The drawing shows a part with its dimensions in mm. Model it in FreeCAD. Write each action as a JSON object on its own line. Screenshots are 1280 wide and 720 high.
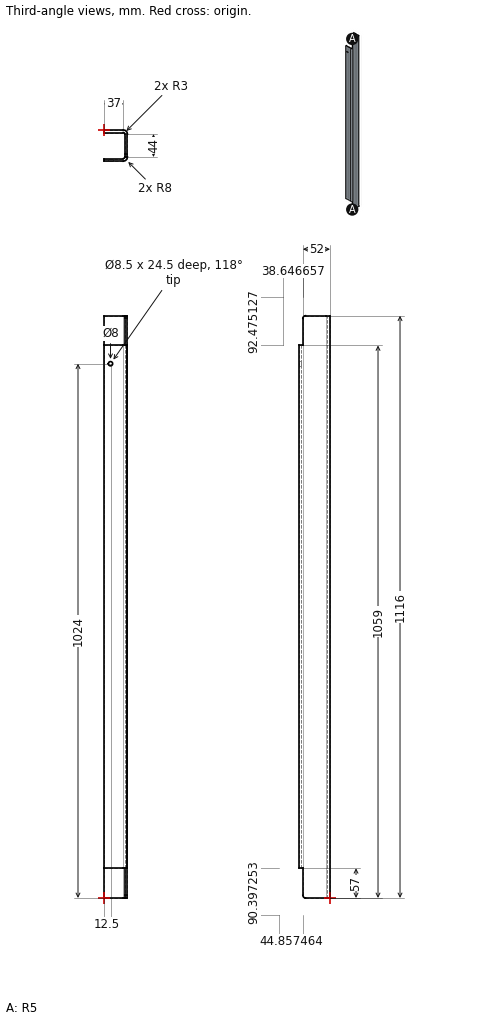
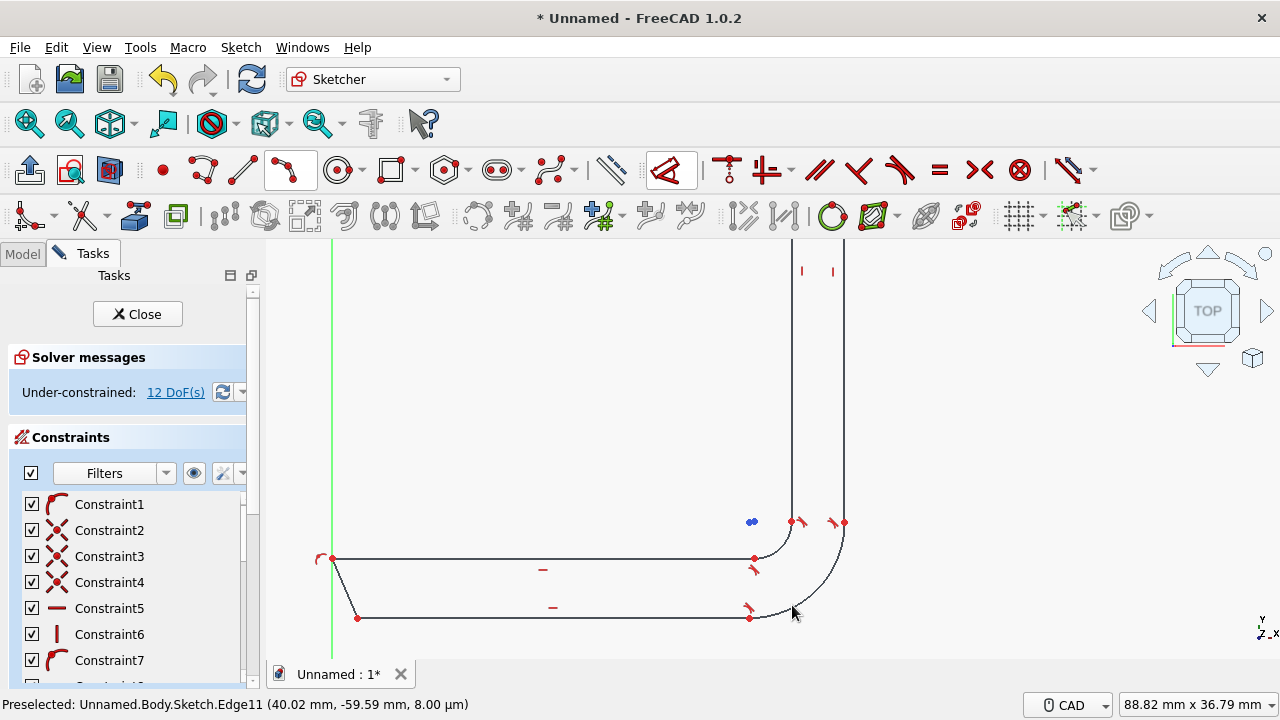
{"action": "left_click", "coordinate": [844, 372]}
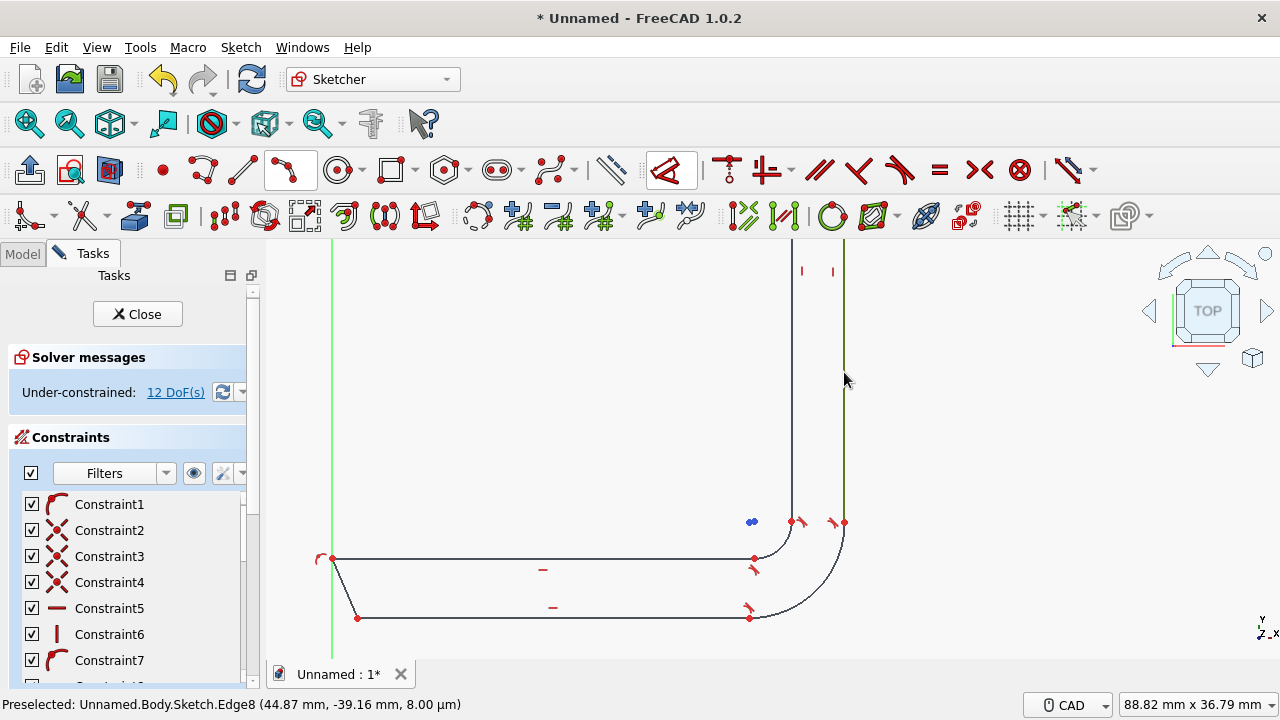
{"action": "scroll", "coordinate": [772, 554], "scroll_direction": "down", "scroll_amount": 5}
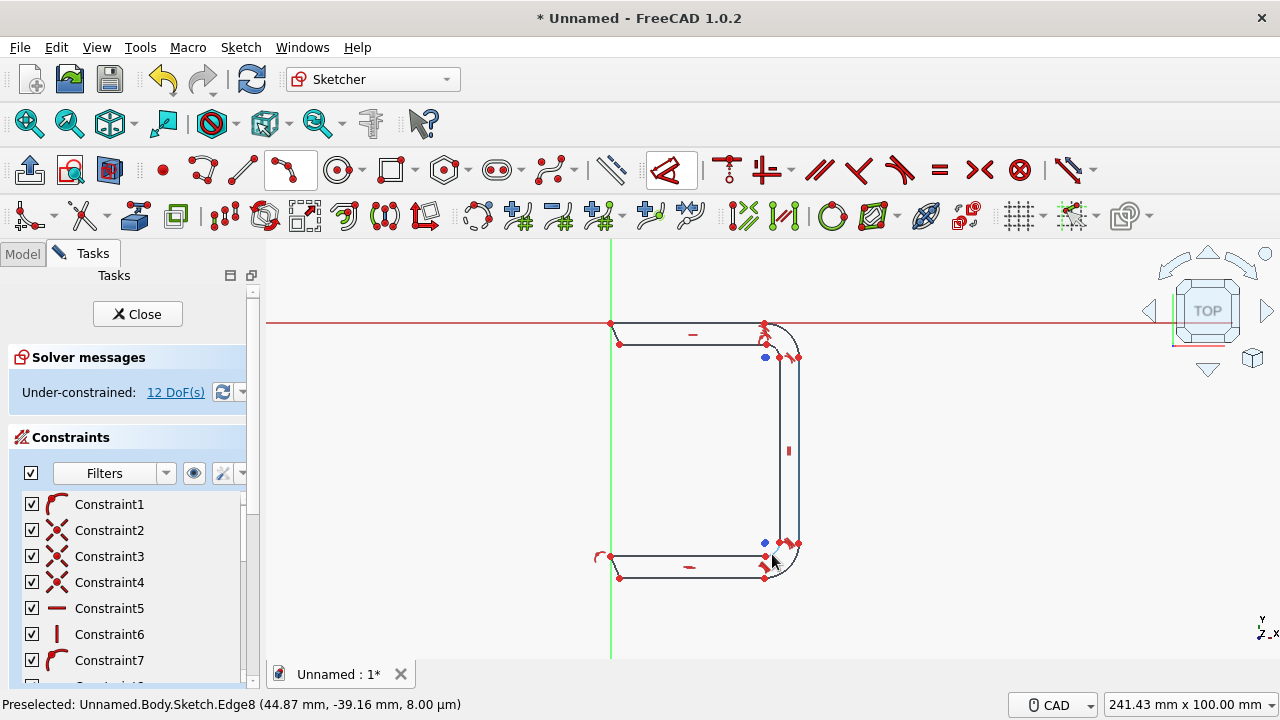
{"action": "left_click", "coordinate": [795, 342]}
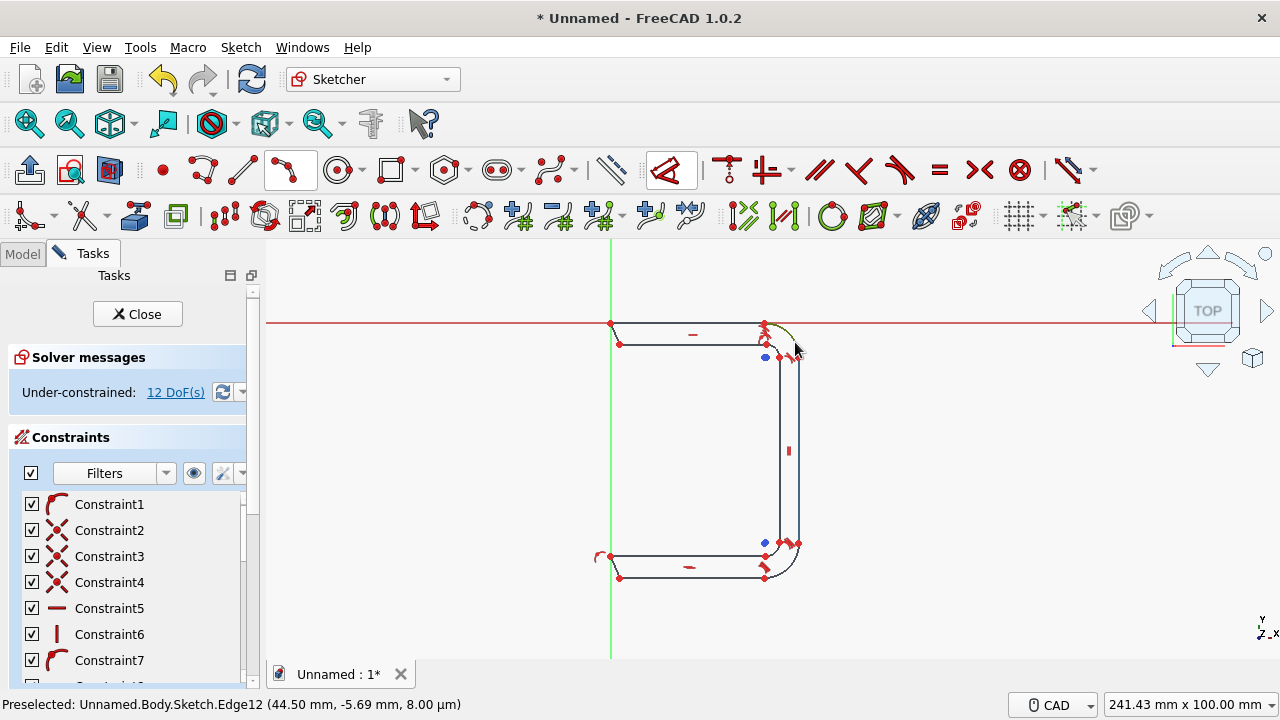
{"action": "key", "text": "t"}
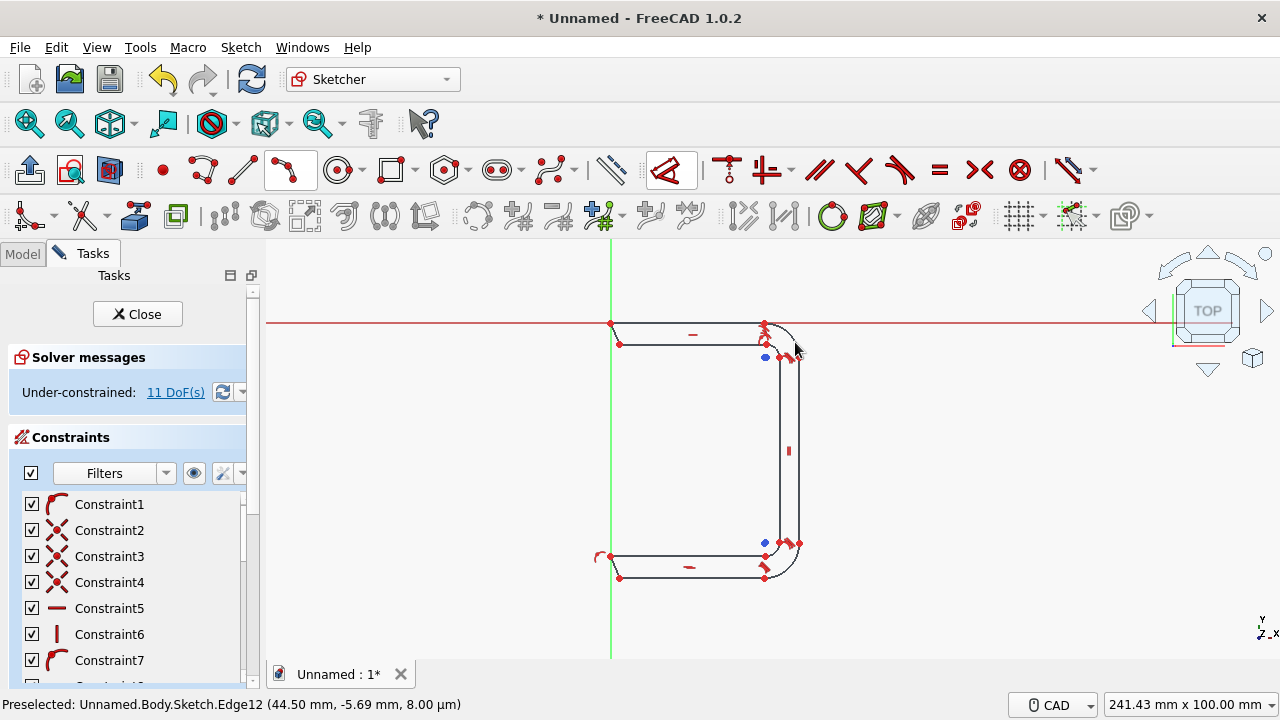
{"action": "scroll", "coordinate": [614, 332], "scroll_direction": "up", "scroll_amount": 3}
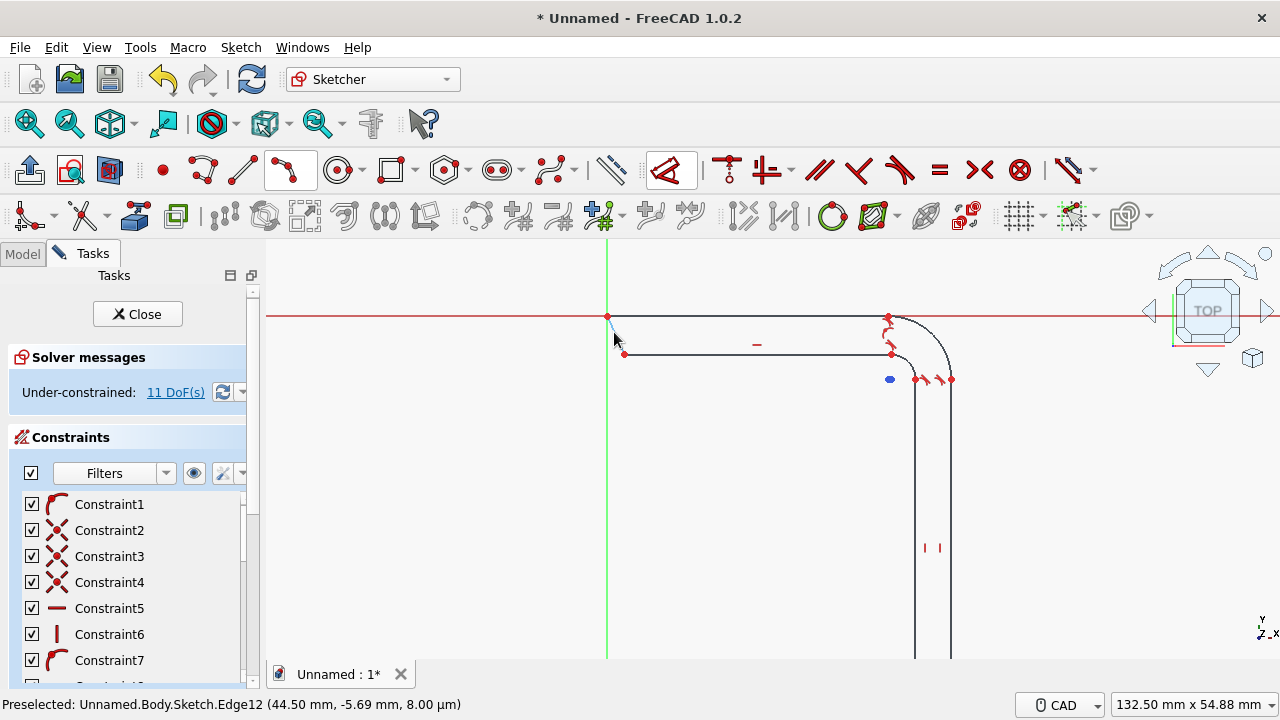
{"action": "left_click", "coordinate": [614, 332]}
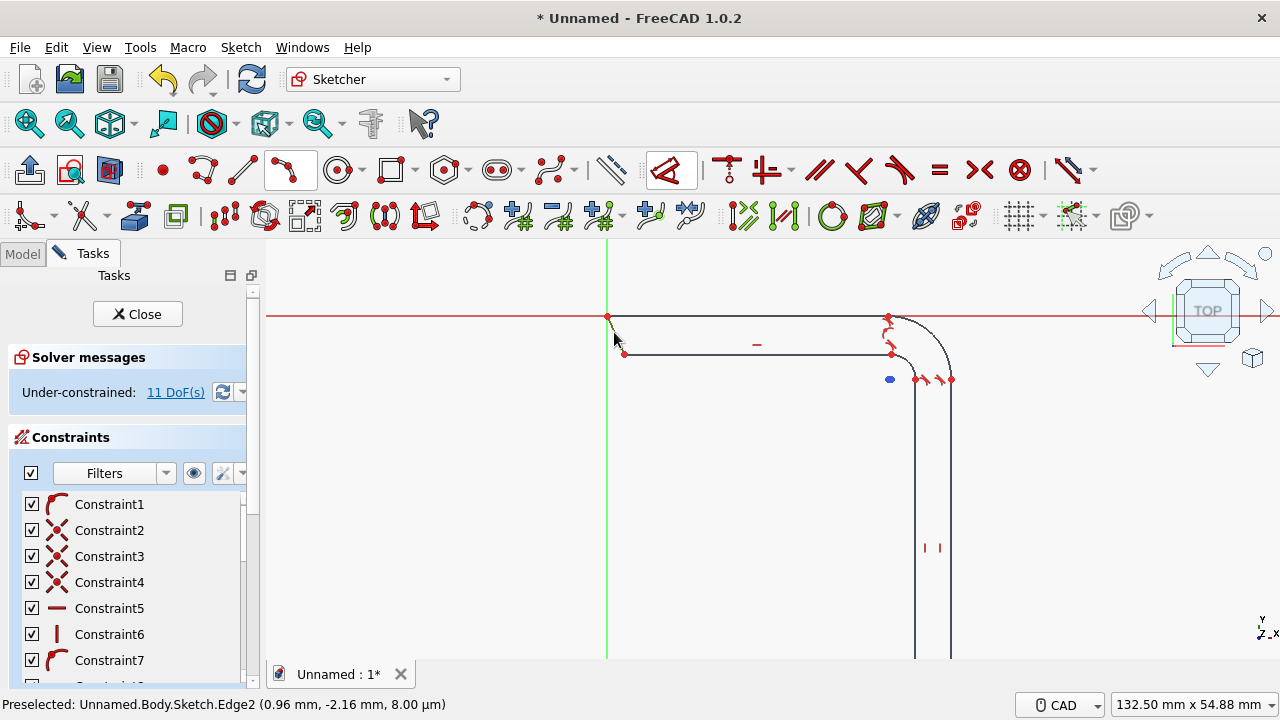
{"action": "key", "text": "v"}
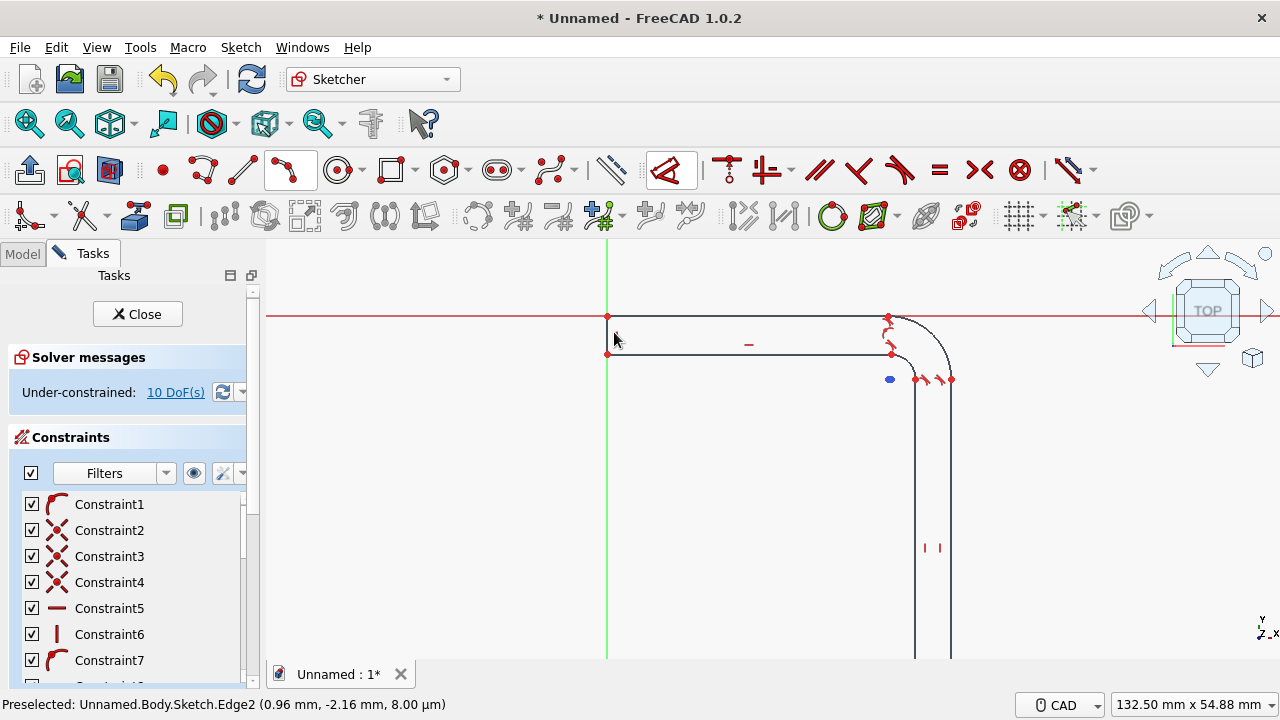
{"action": "scroll", "coordinate": [613, 331], "scroll_direction": "down", "scroll_amount": 3}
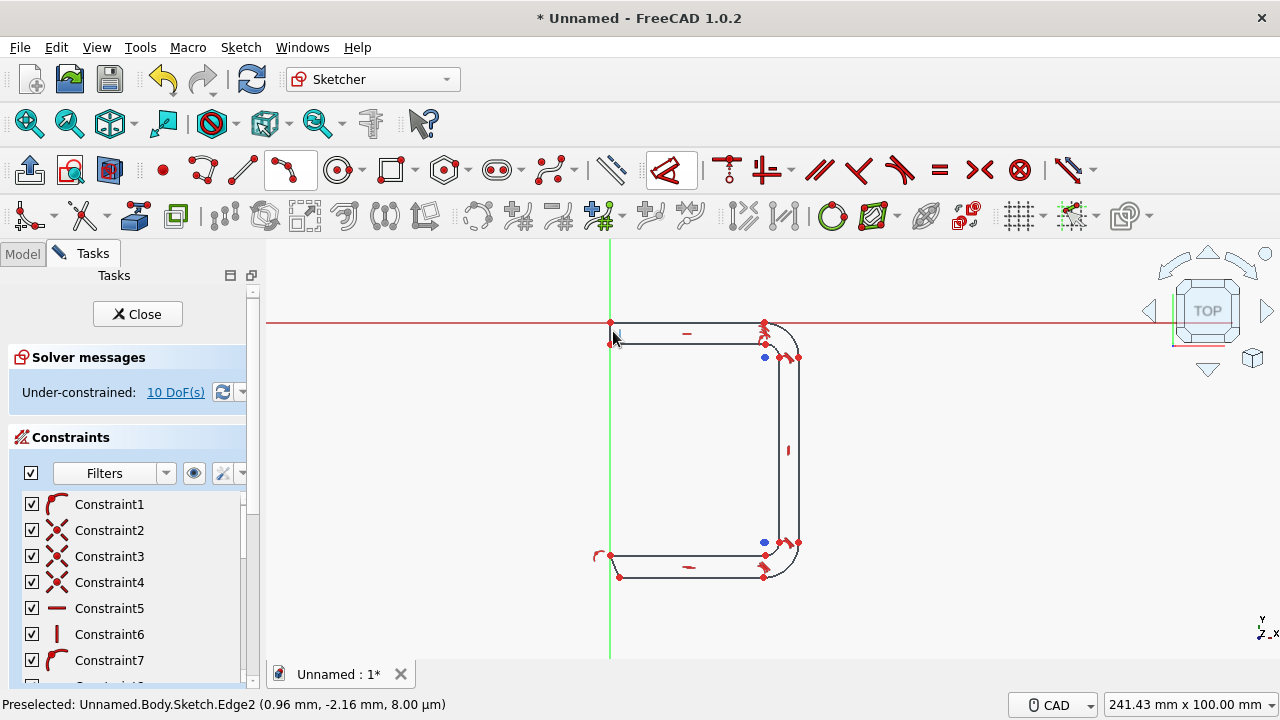
{"action": "scroll", "coordinate": [617, 571], "scroll_direction": "up", "scroll_amount": 4}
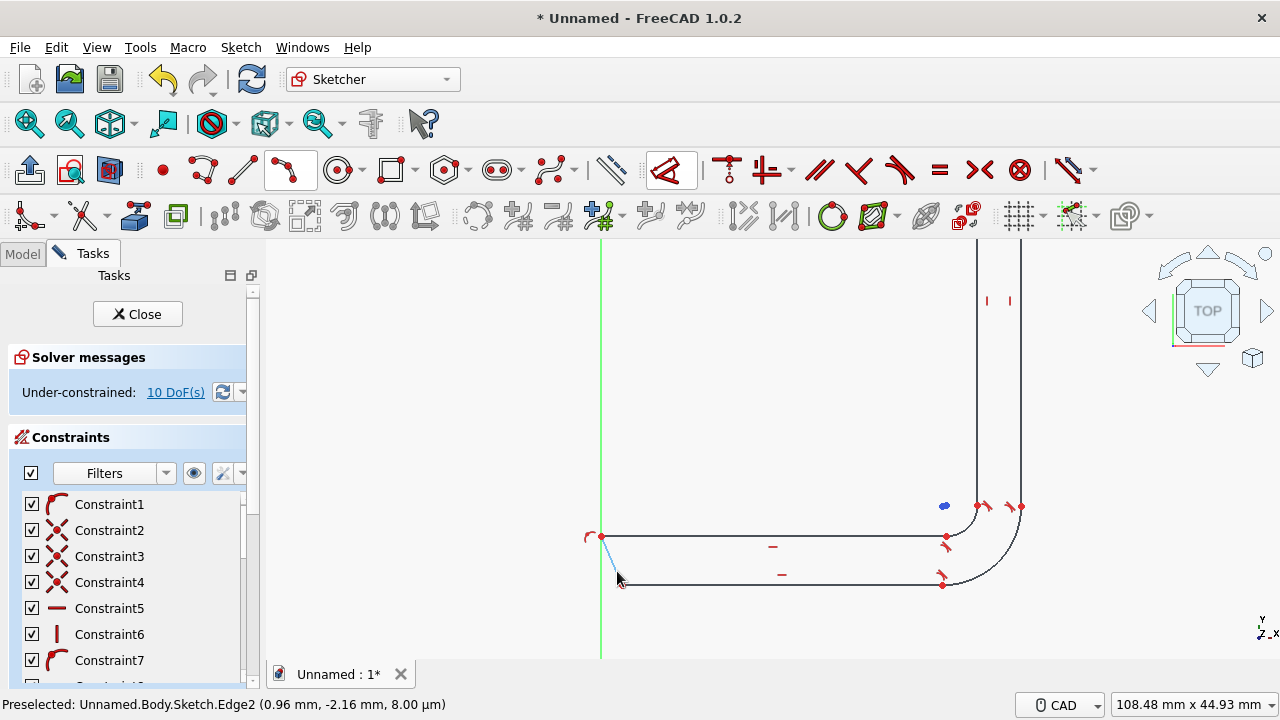
{"action": "left_click", "coordinate": [616, 570]}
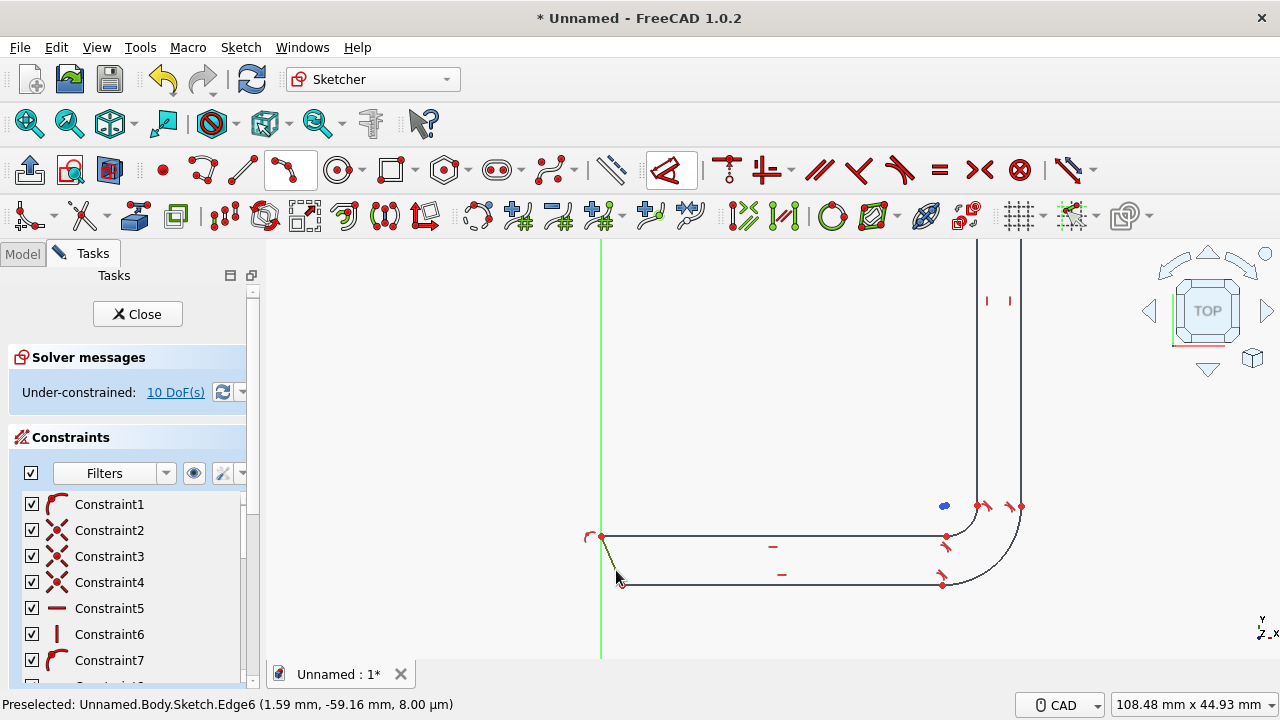
{"action": "key", "text": "v"}